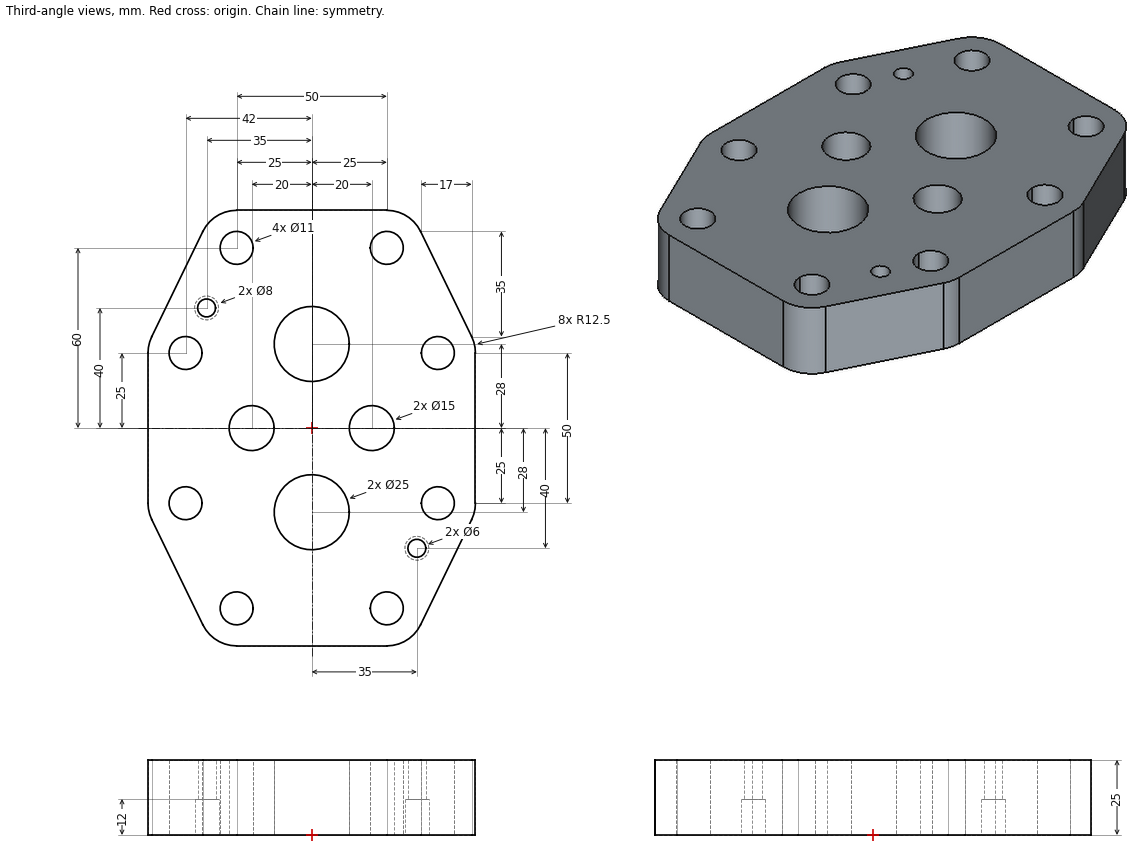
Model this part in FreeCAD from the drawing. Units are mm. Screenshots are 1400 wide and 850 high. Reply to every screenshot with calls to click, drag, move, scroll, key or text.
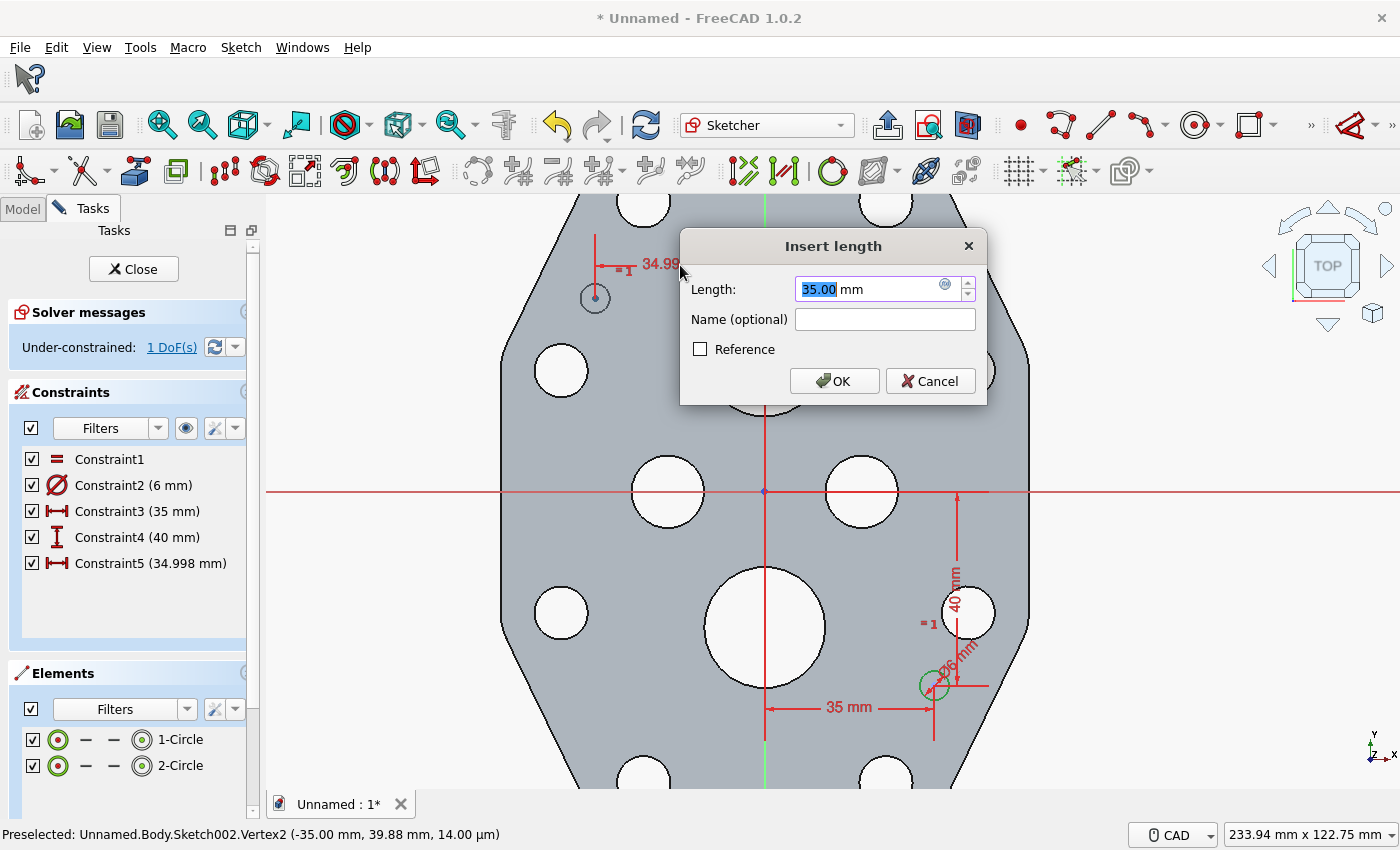
text(35)
key(Return)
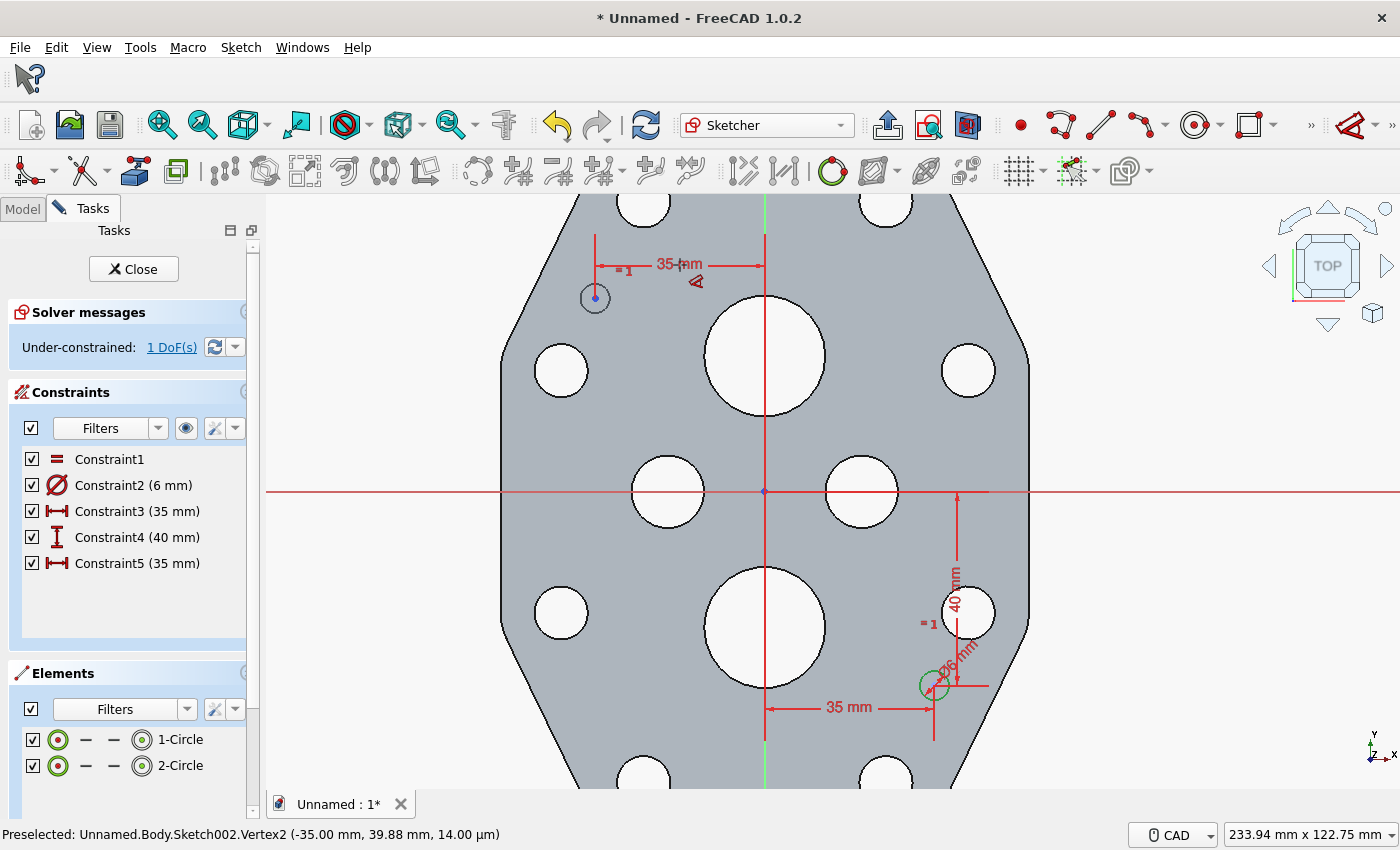
click(595, 299)
click(561, 395)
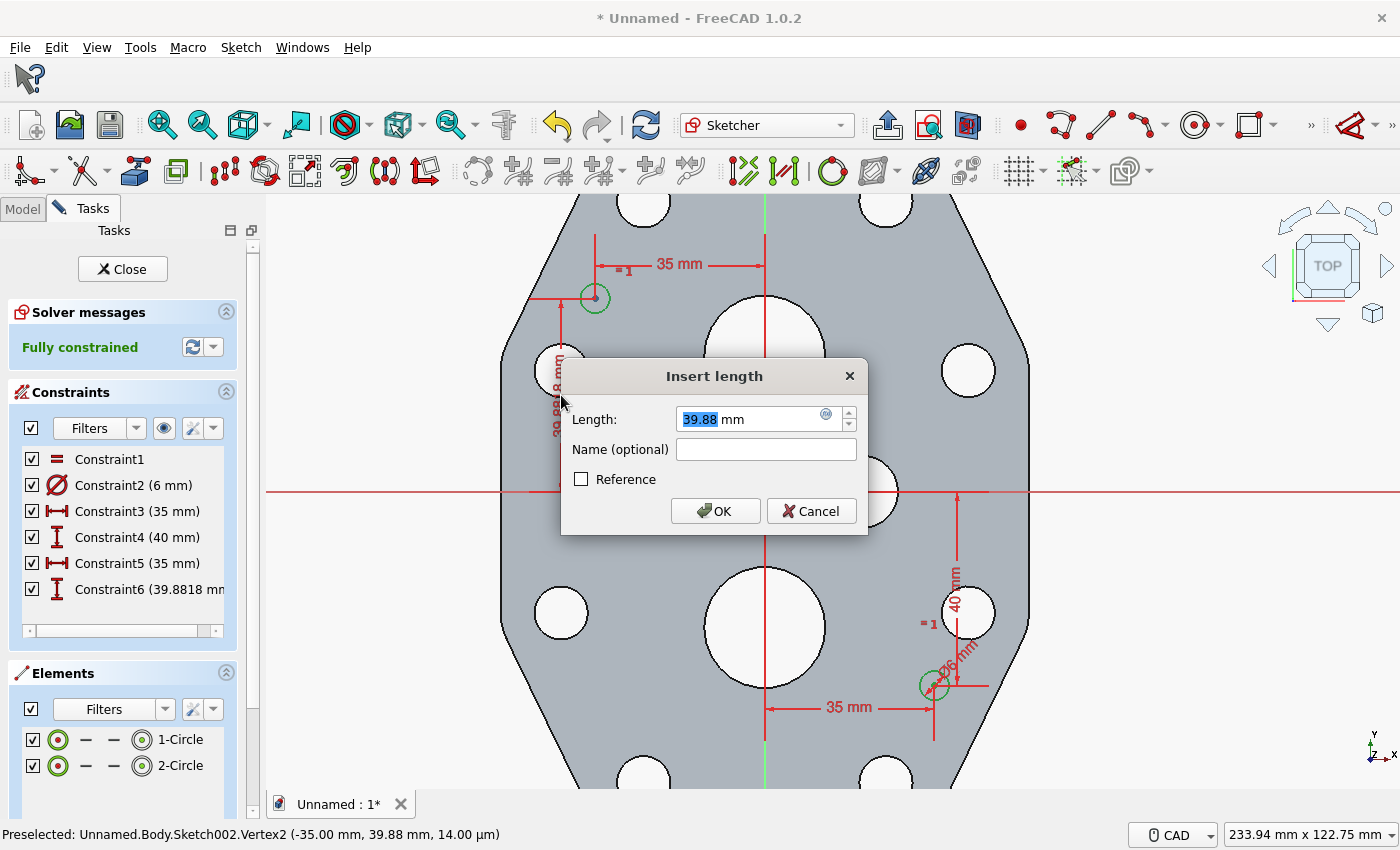
text(40)
key(Return)
key(Escape)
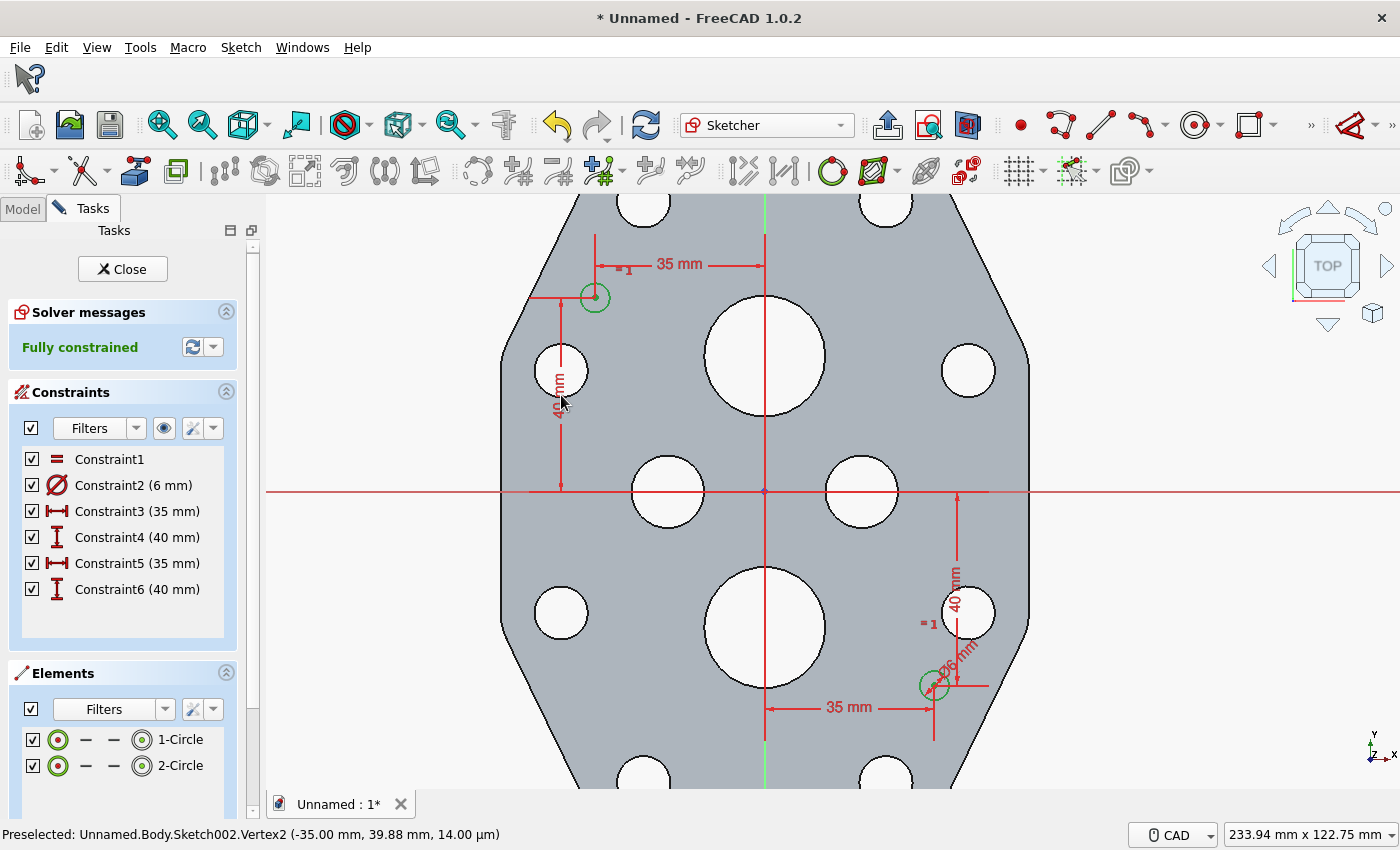
click(123, 269)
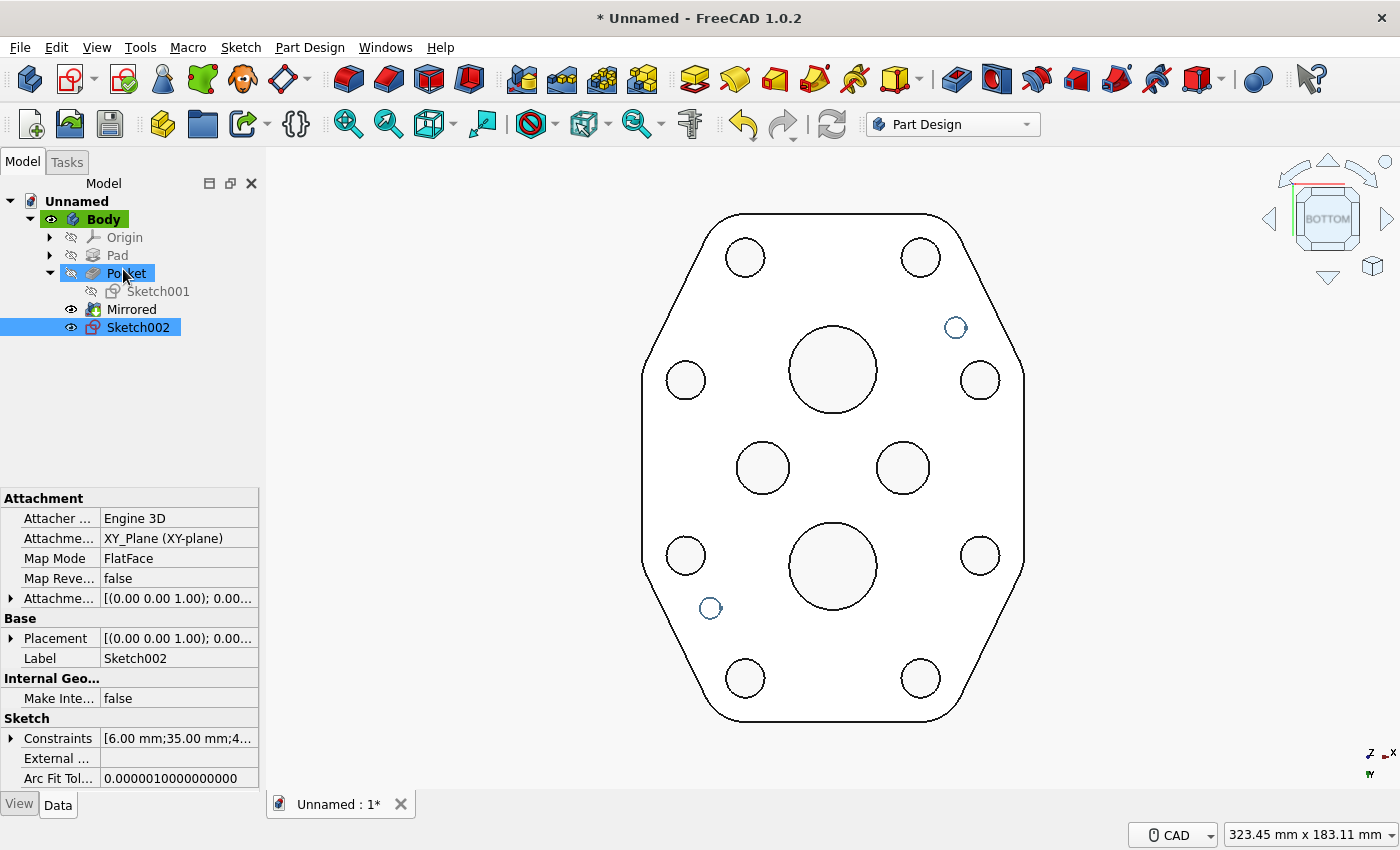
click(958, 80)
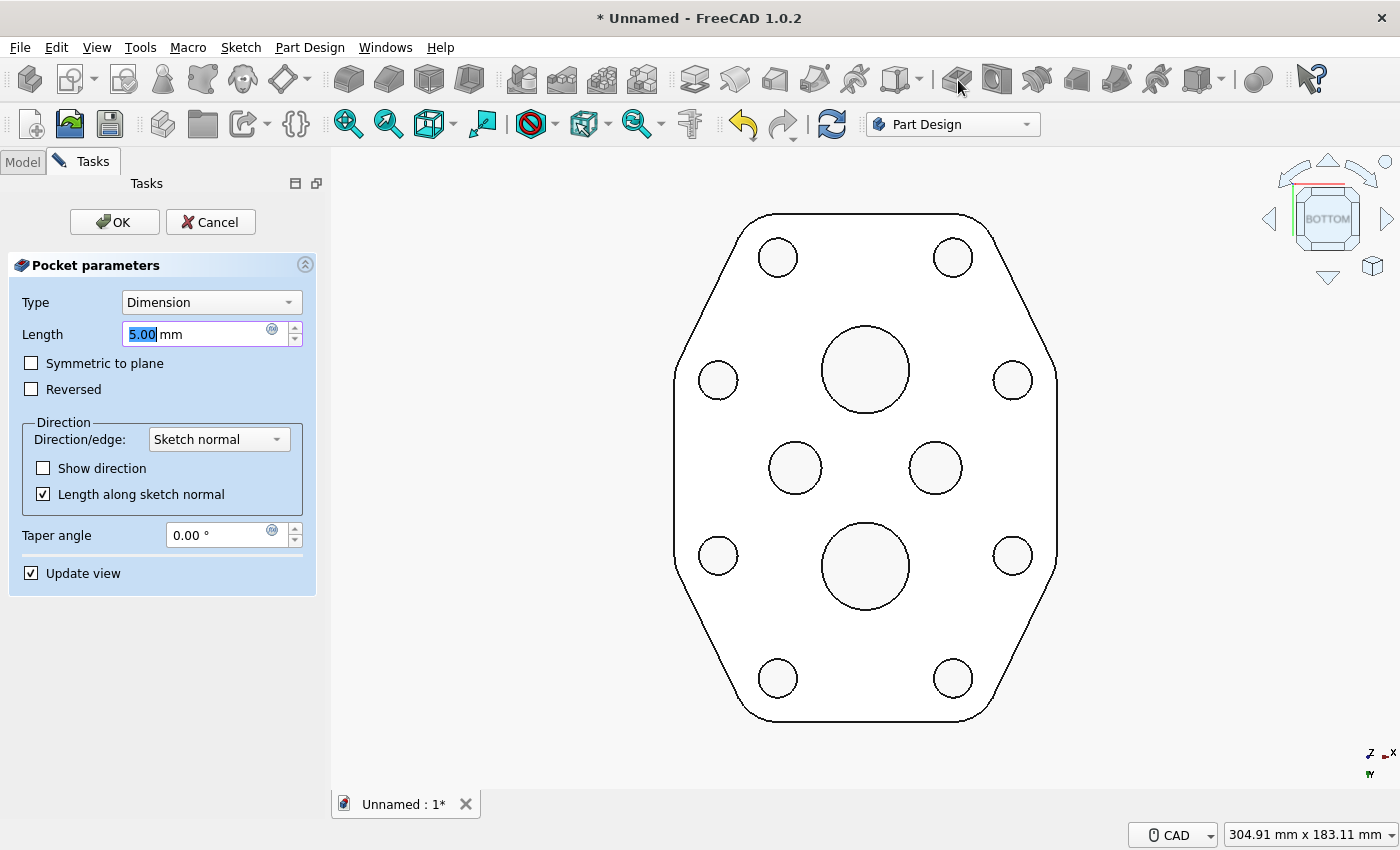
click(212, 302)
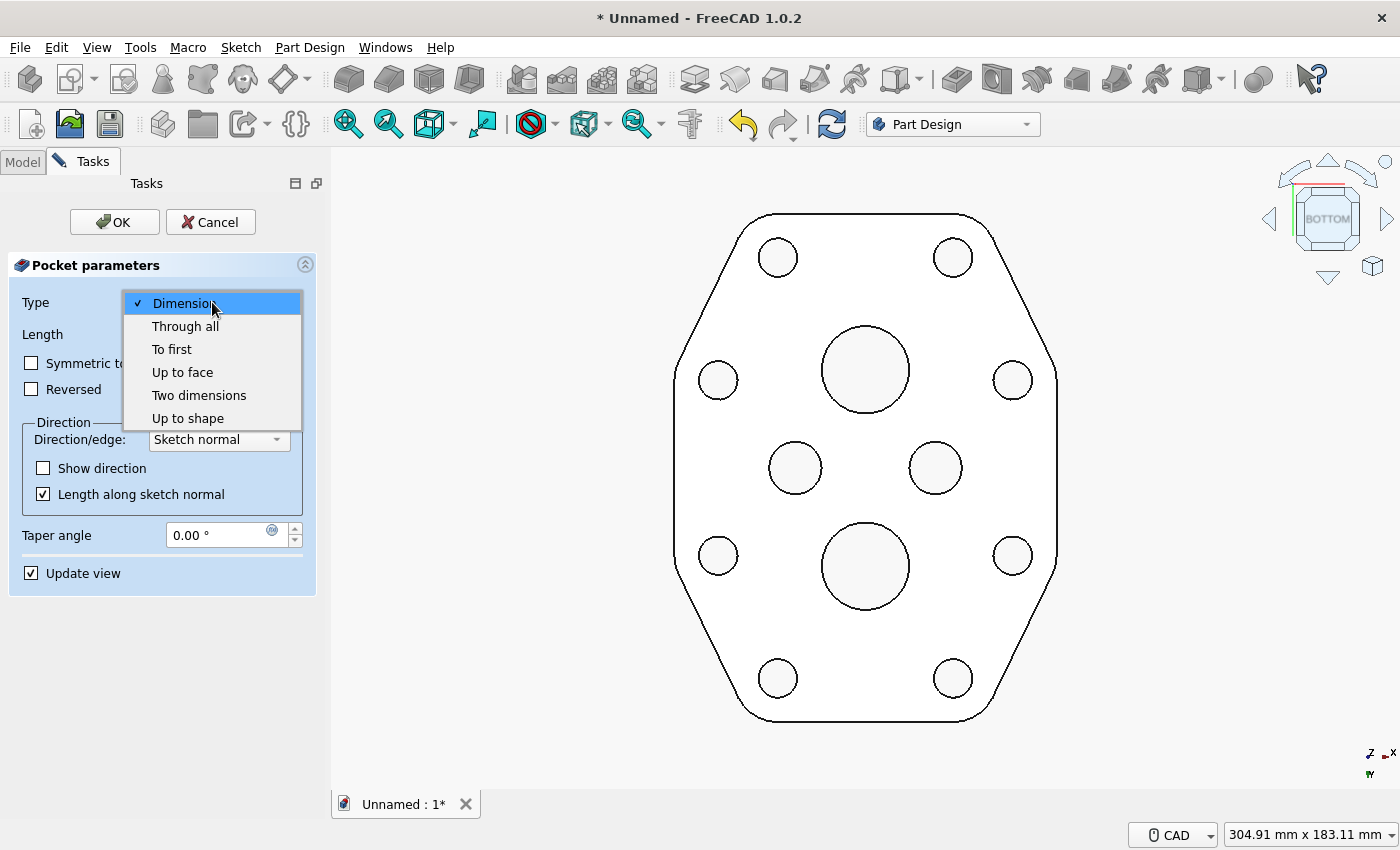
click(212, 326)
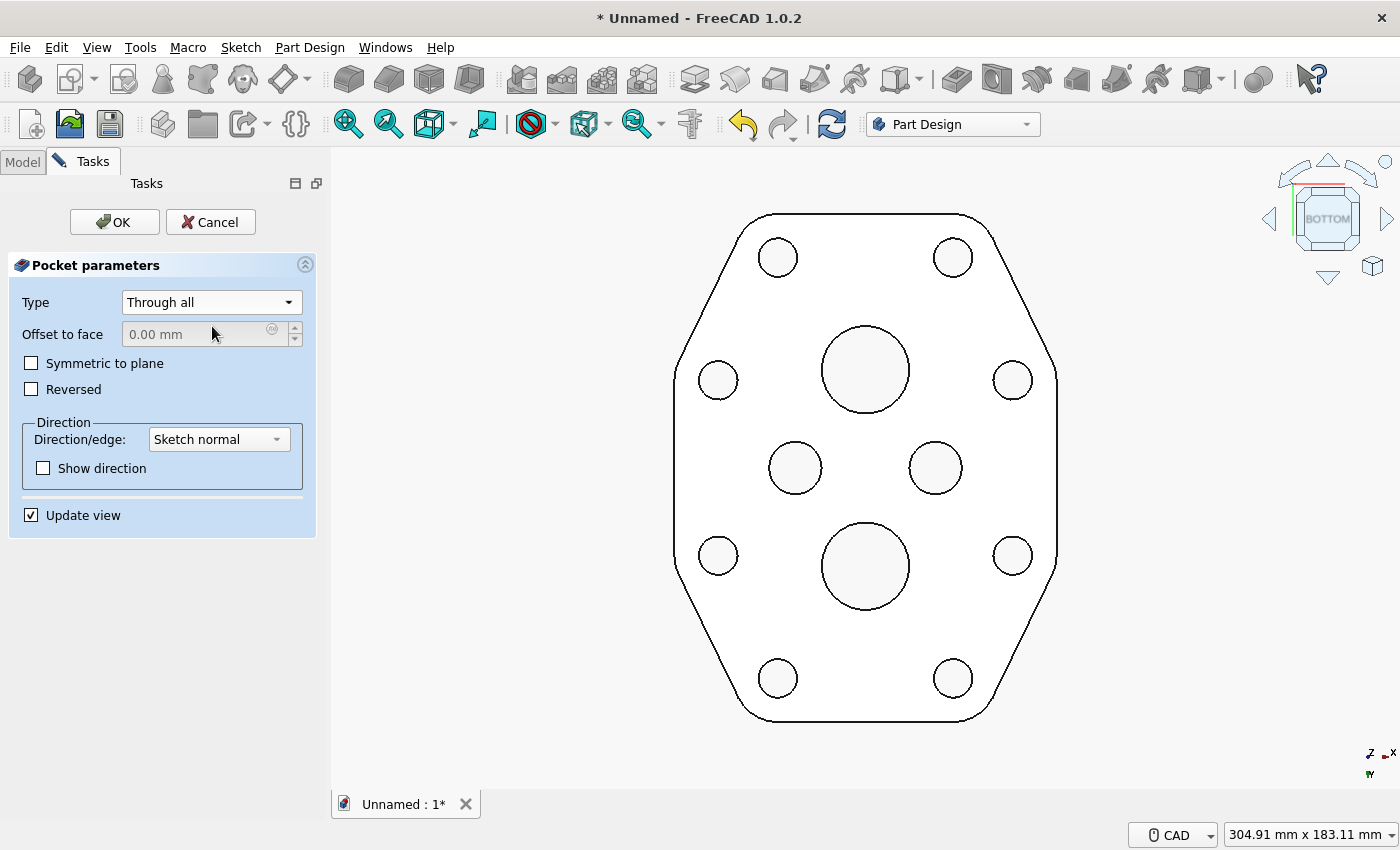
click(30, 389)